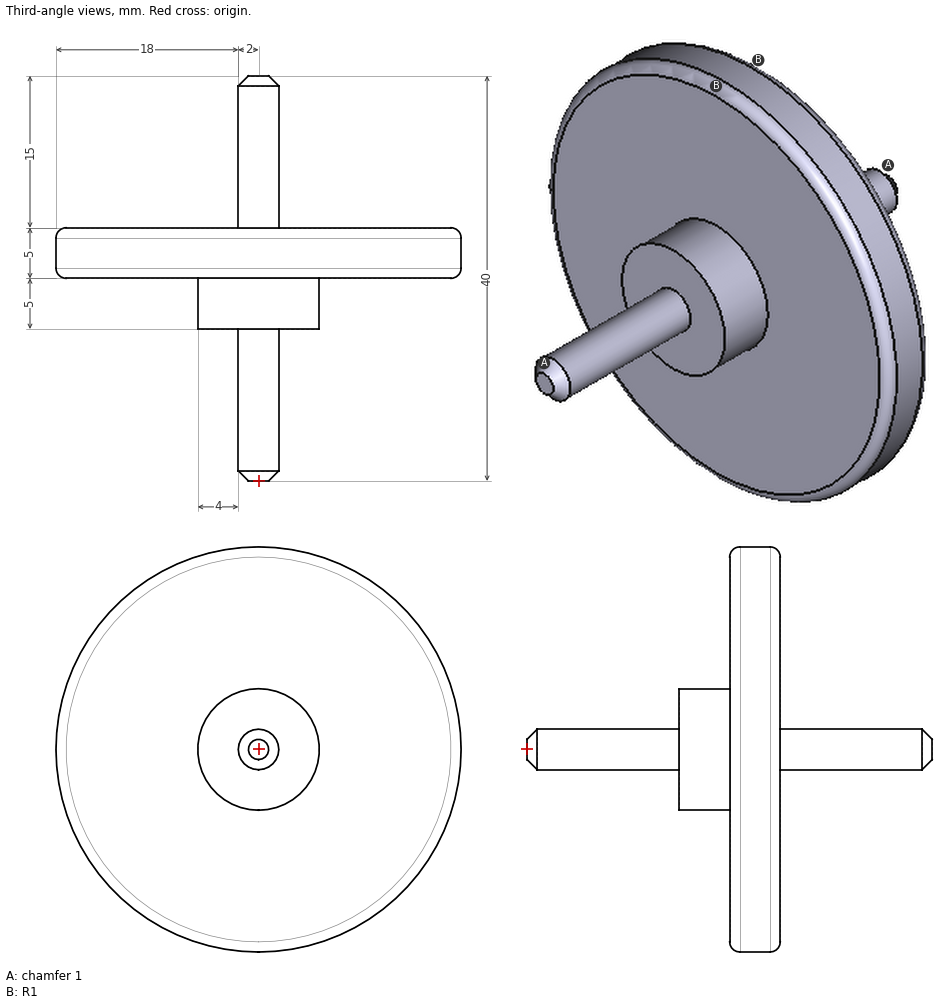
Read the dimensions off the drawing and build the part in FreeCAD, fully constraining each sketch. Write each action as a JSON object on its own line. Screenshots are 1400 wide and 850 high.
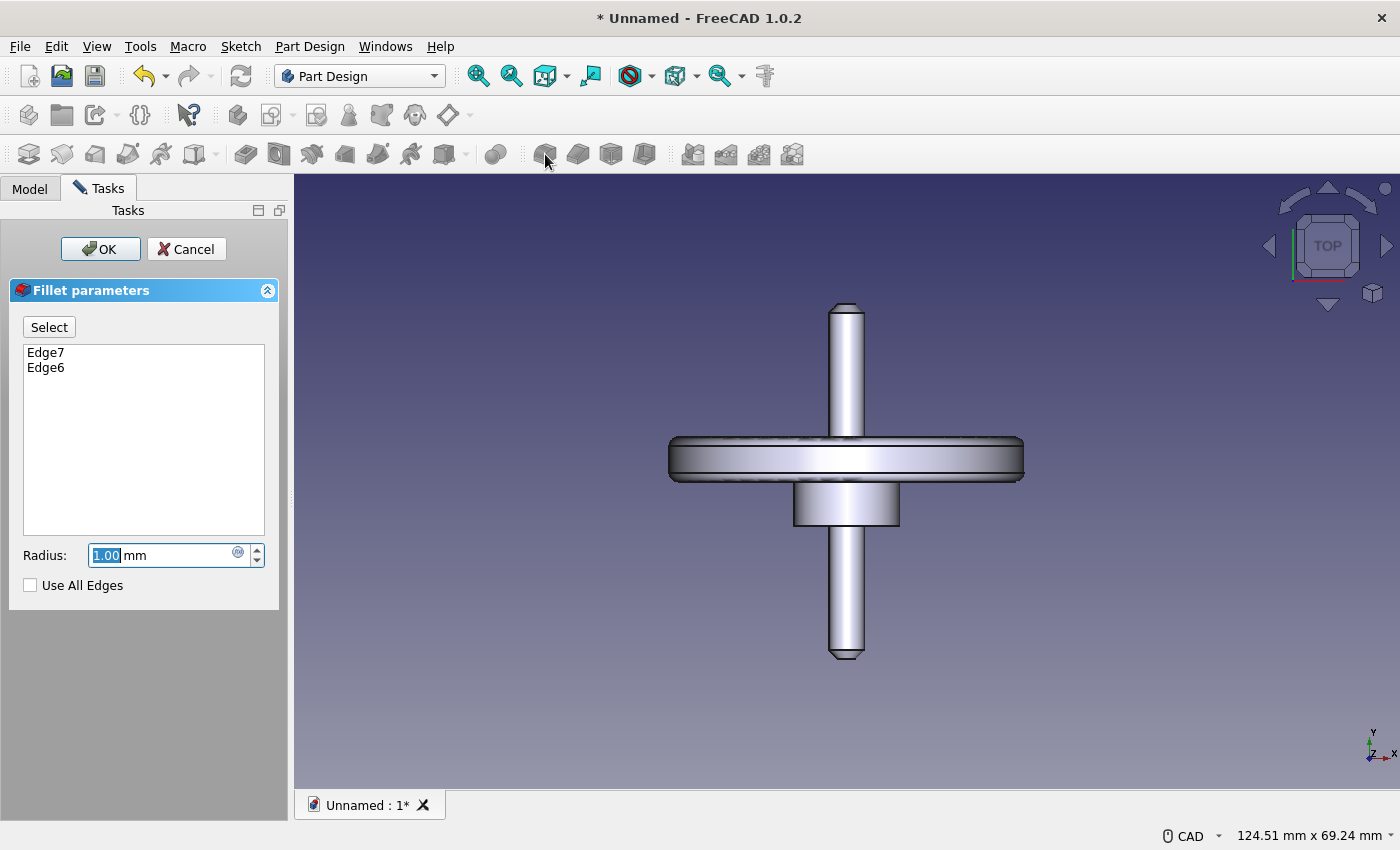
{"action": "type", "text": "1"}
{"action": "key", "text": "Tab"}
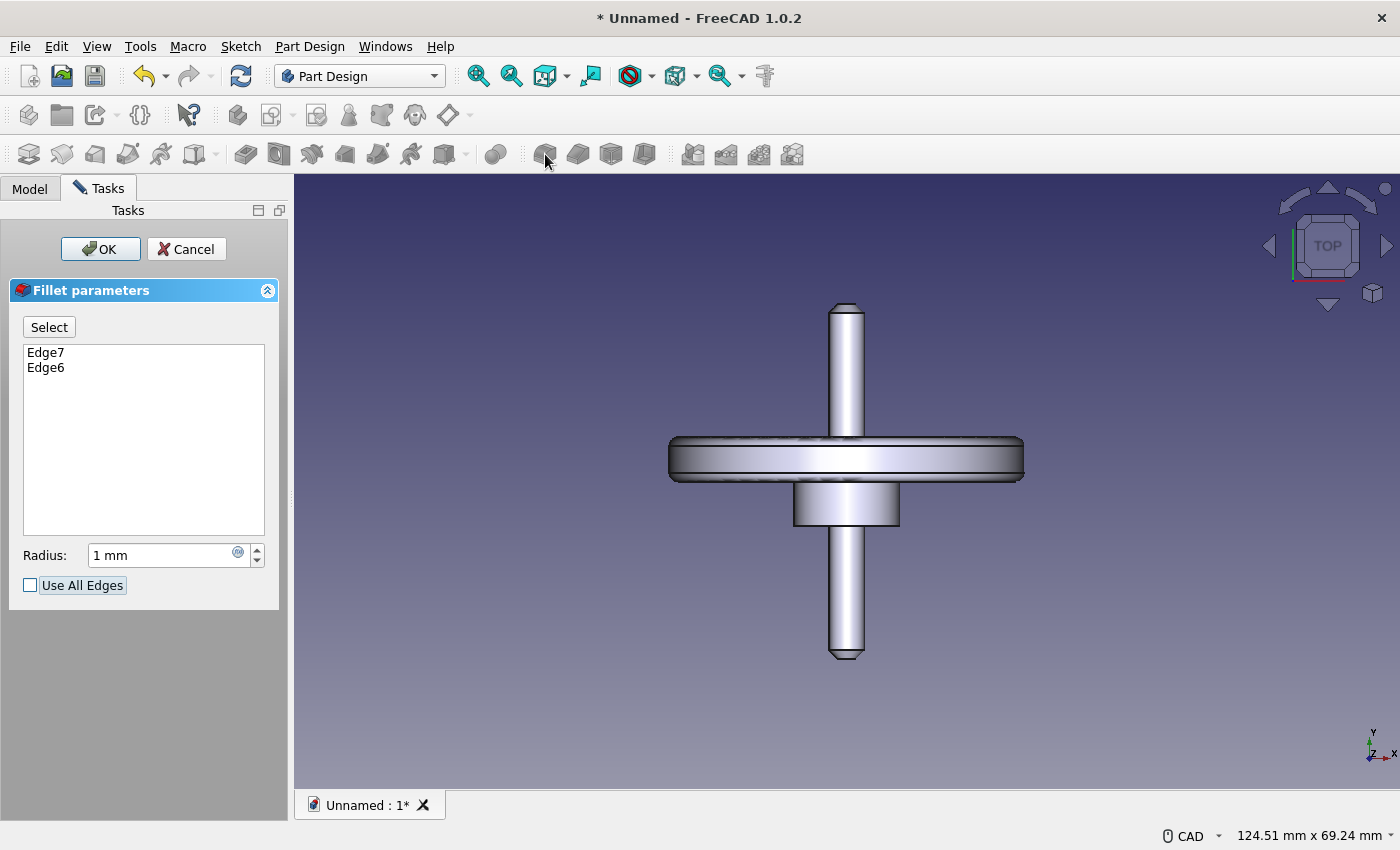
{"action": "left_click", "coordinate": [101, 249]}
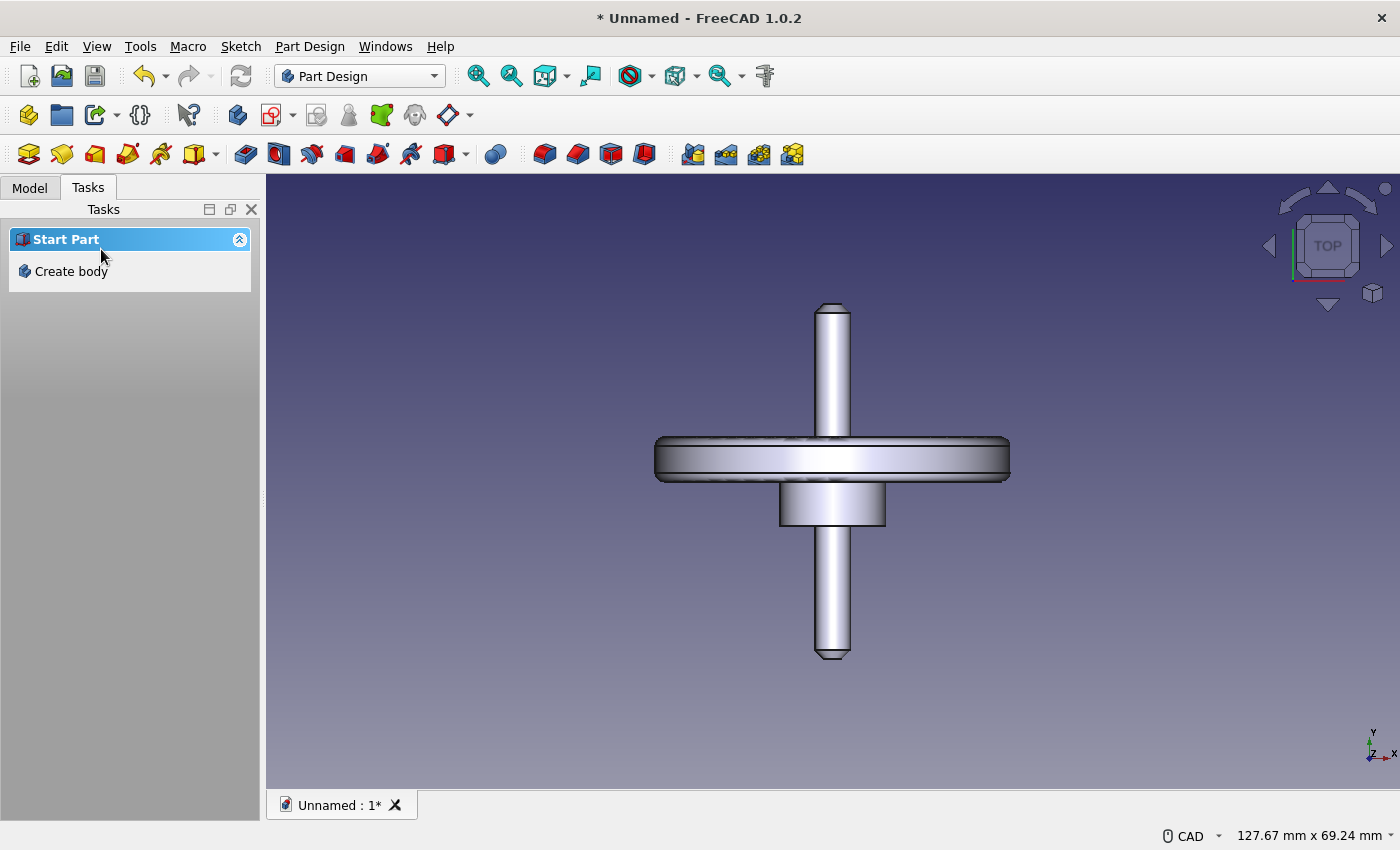
{"action": "key", "text": "0"}